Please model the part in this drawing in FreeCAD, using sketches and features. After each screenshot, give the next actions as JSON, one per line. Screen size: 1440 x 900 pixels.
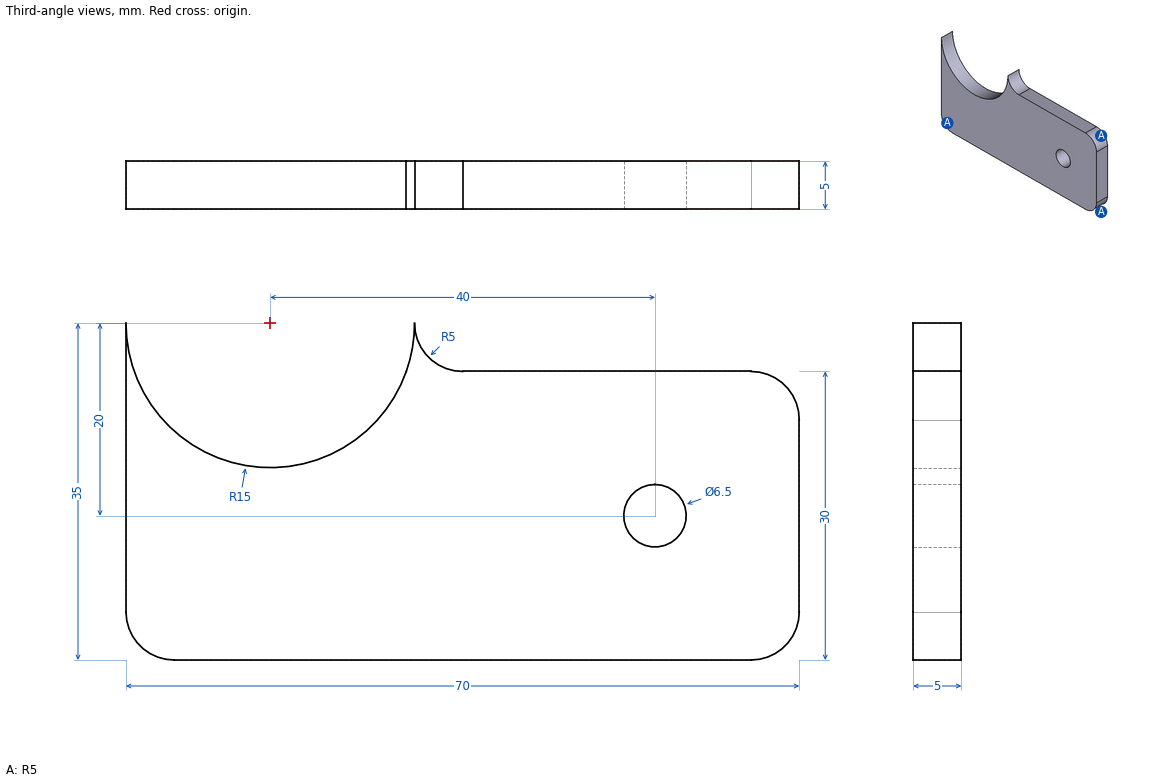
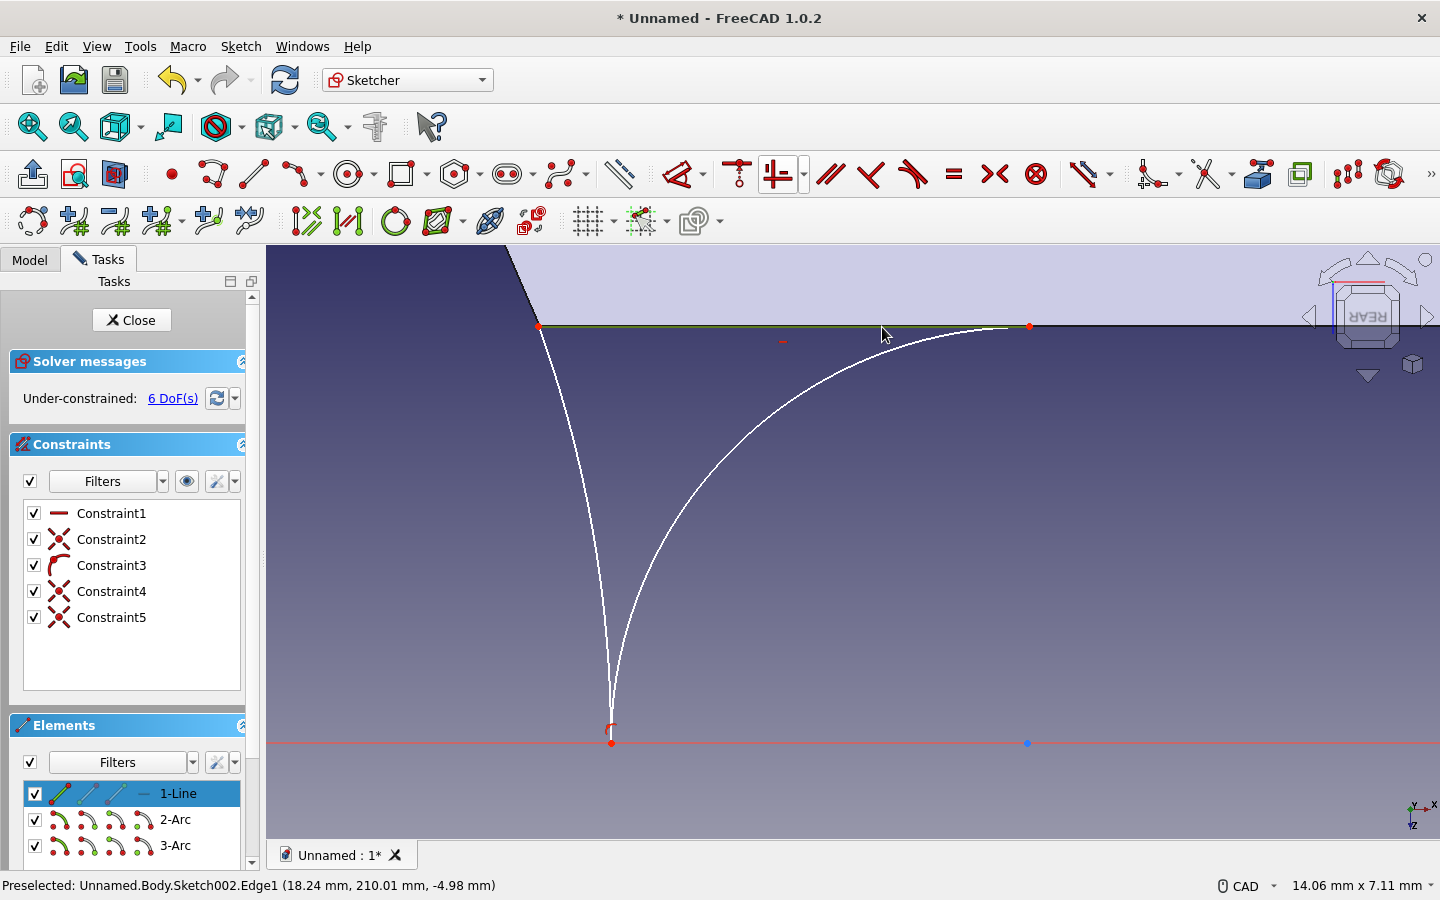
{"action": "left_click", "coordinate": [839, 372]}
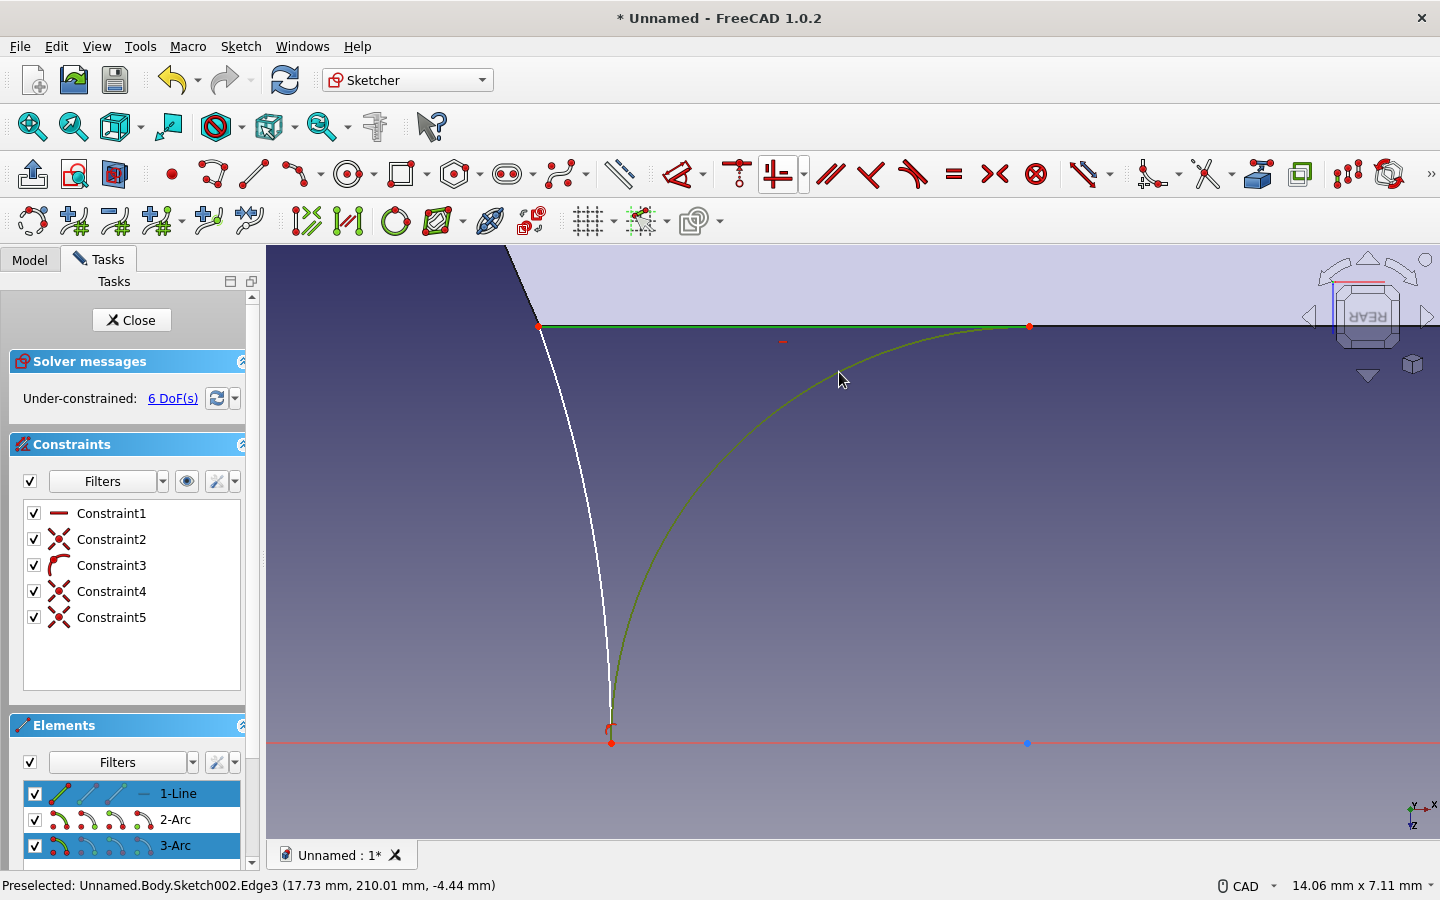
{"action": "left_click", "coordinate": [913, 174]}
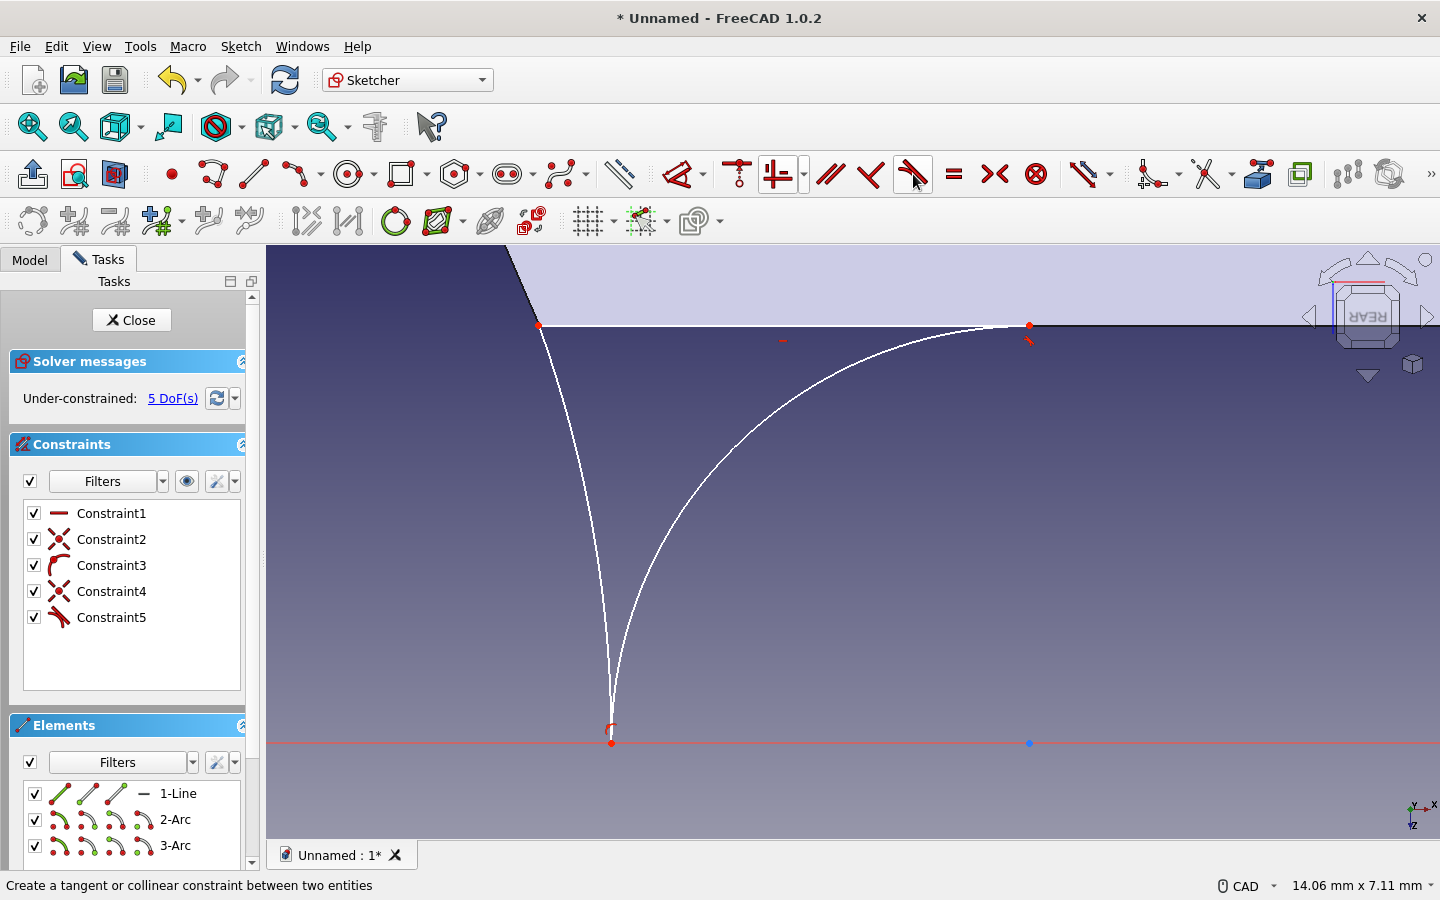
{"action": "left_click", "coordinate": [605, 616]}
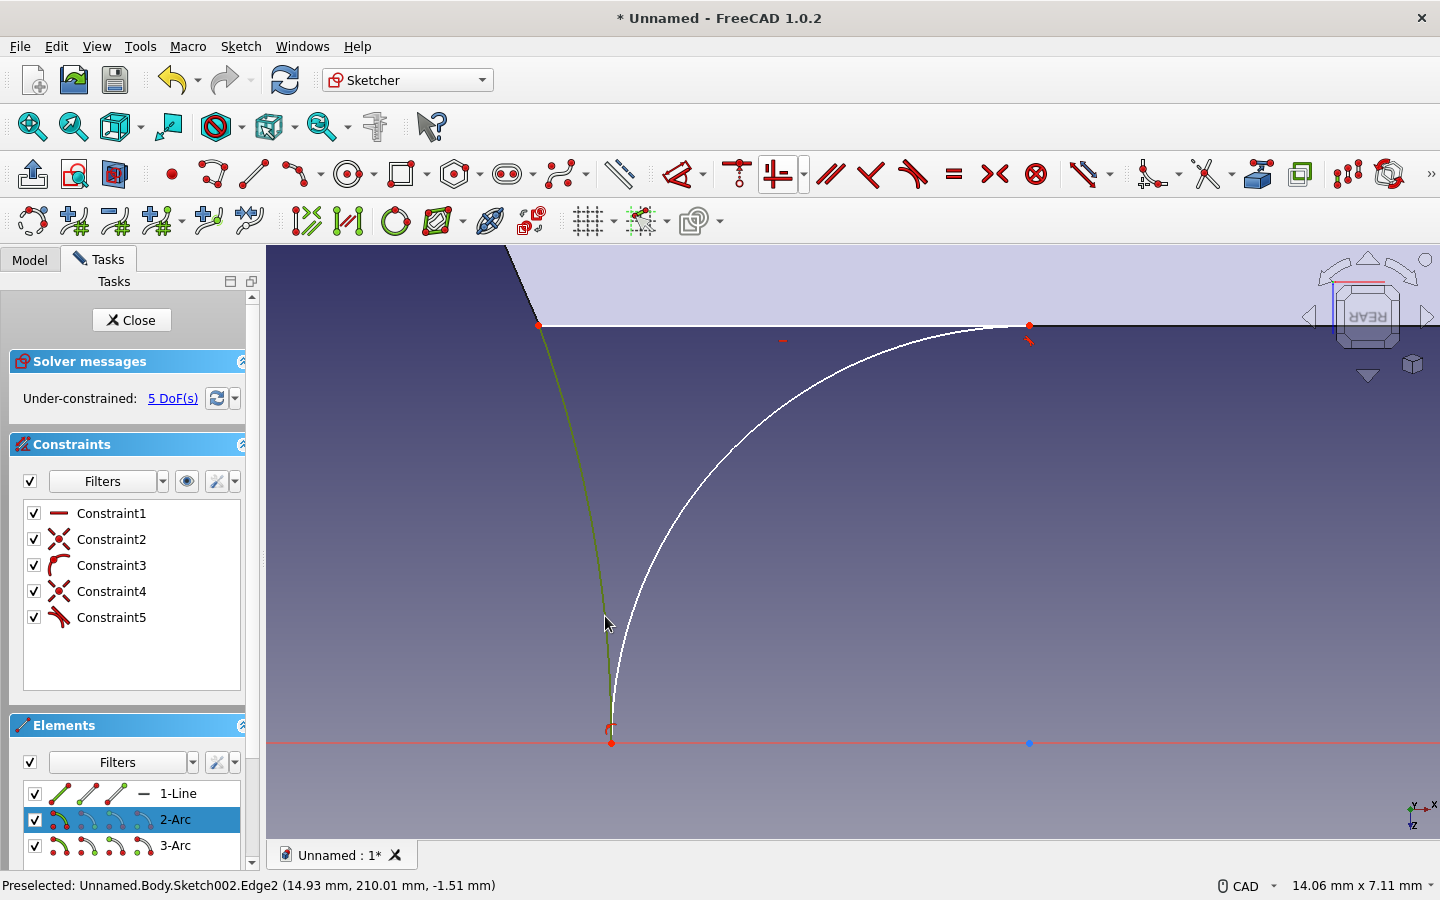
{"action": "left_click", "coordinate": [840, 371]}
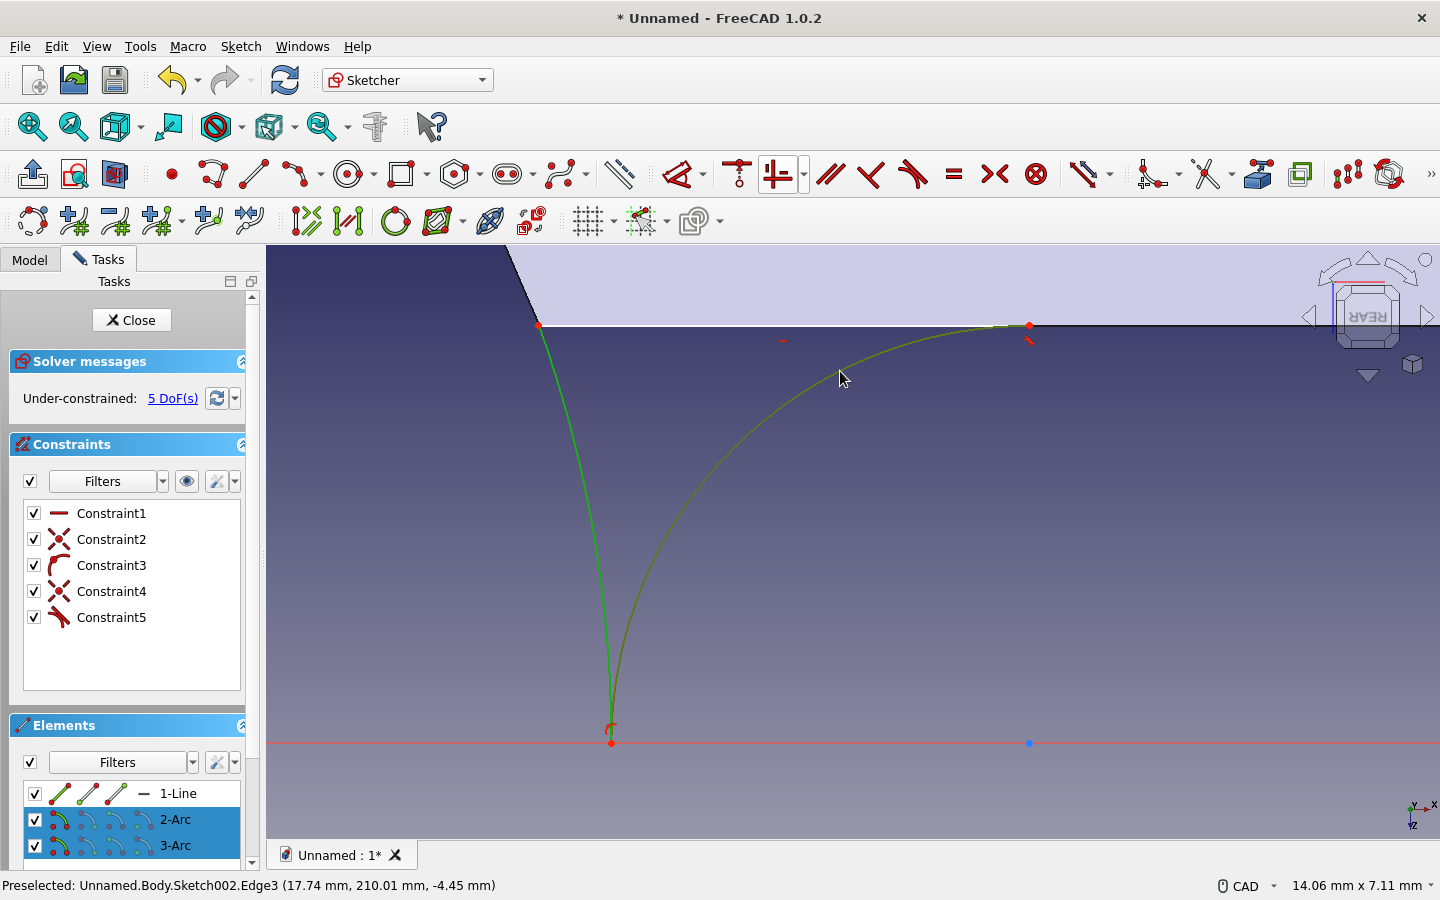
{"action": "left_click", "coordinate": [913, 174]}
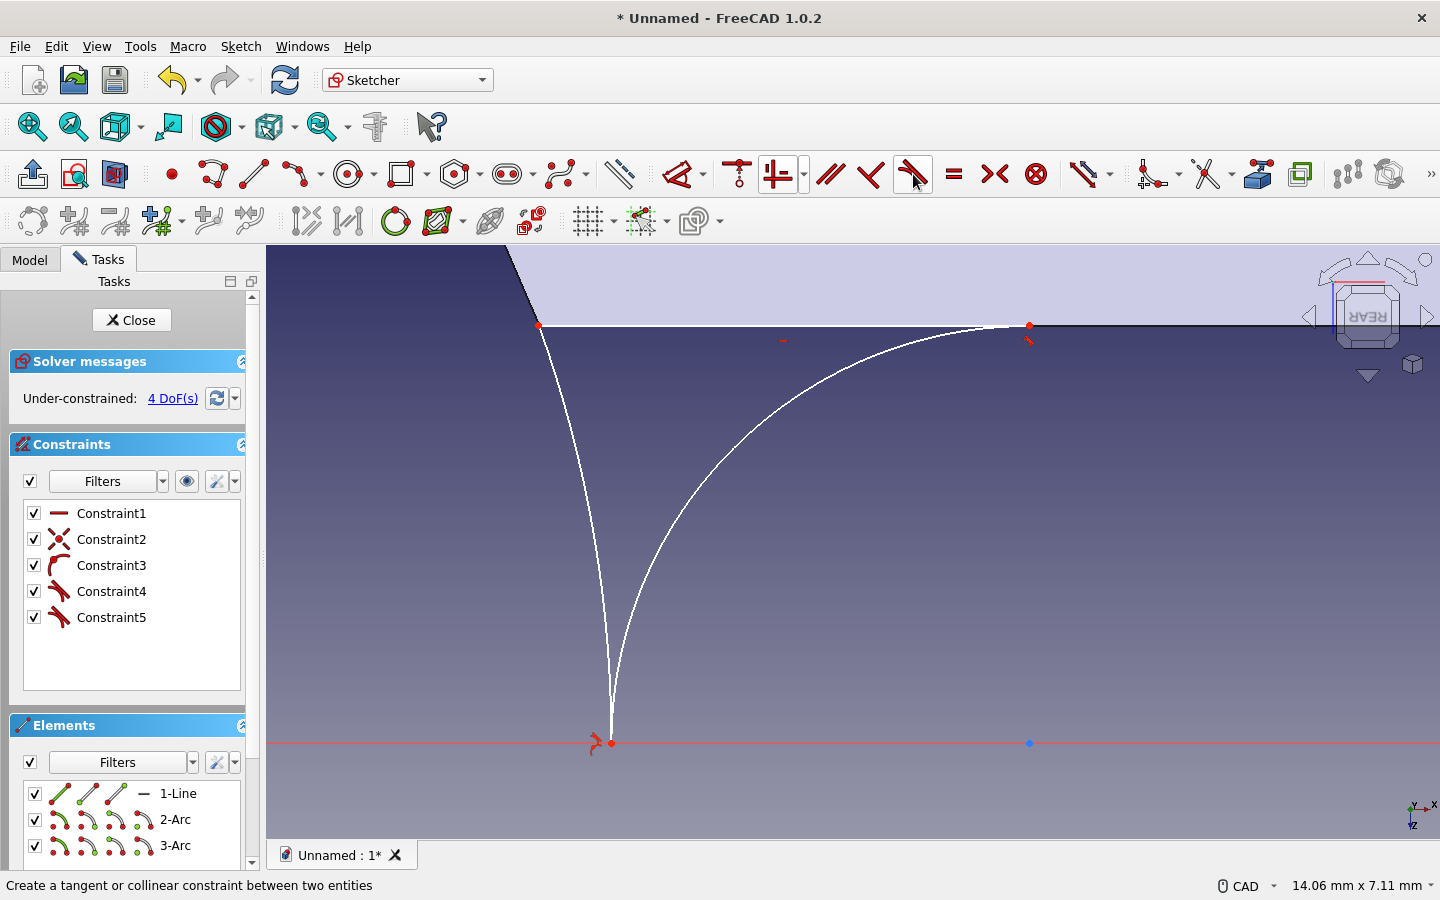
{"action": "scroll", "coordinate": [1262, 548], "scroll_direction": "down", "scroll_amount": 4}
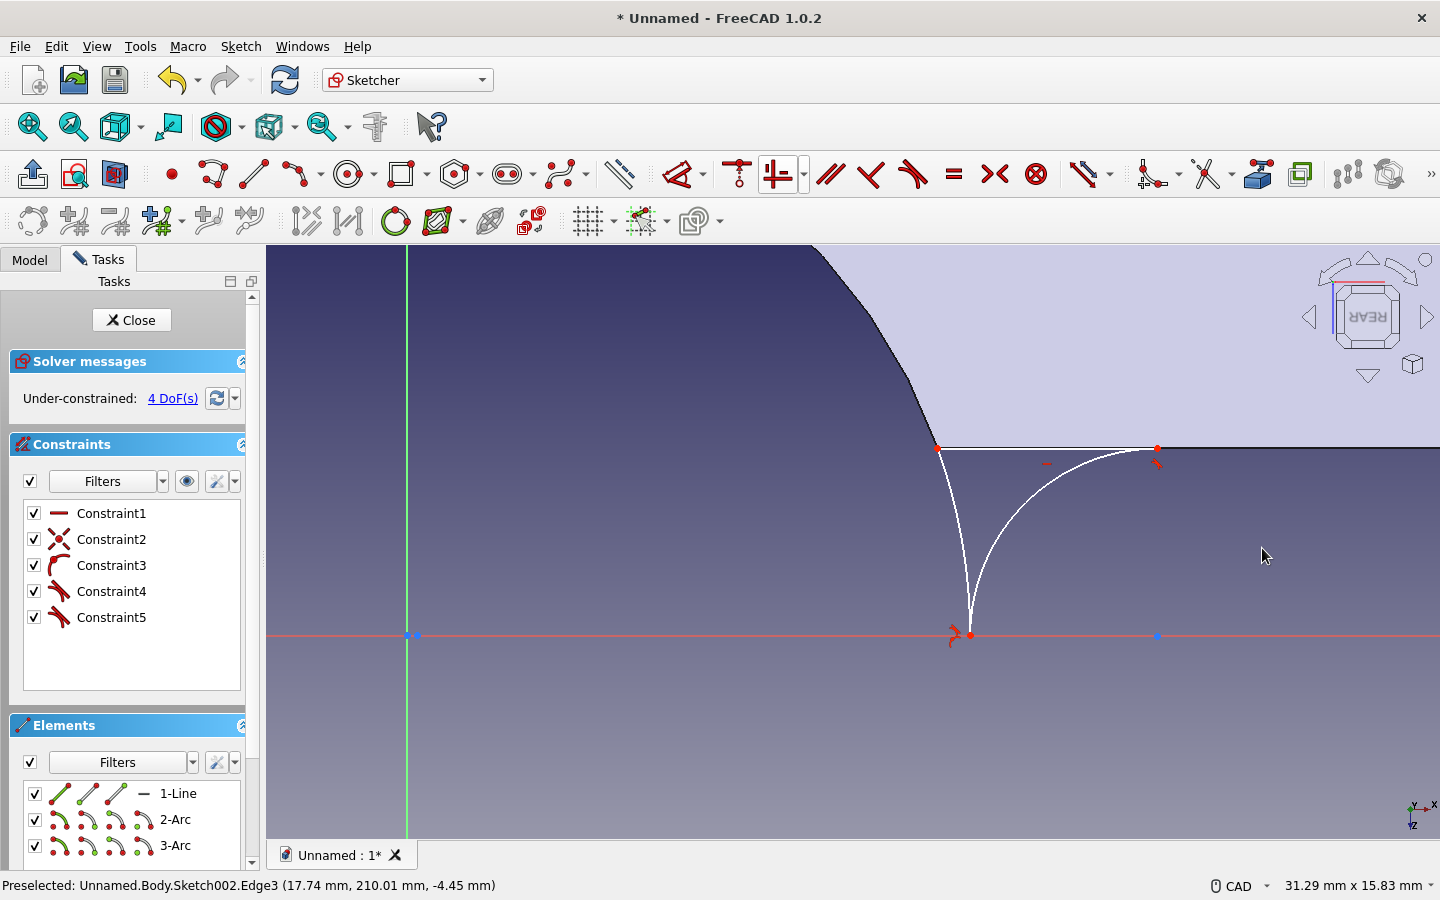
{"action": "left_click_drag", "start_coordinate": [397, 625], "coordinate": [427, 646]}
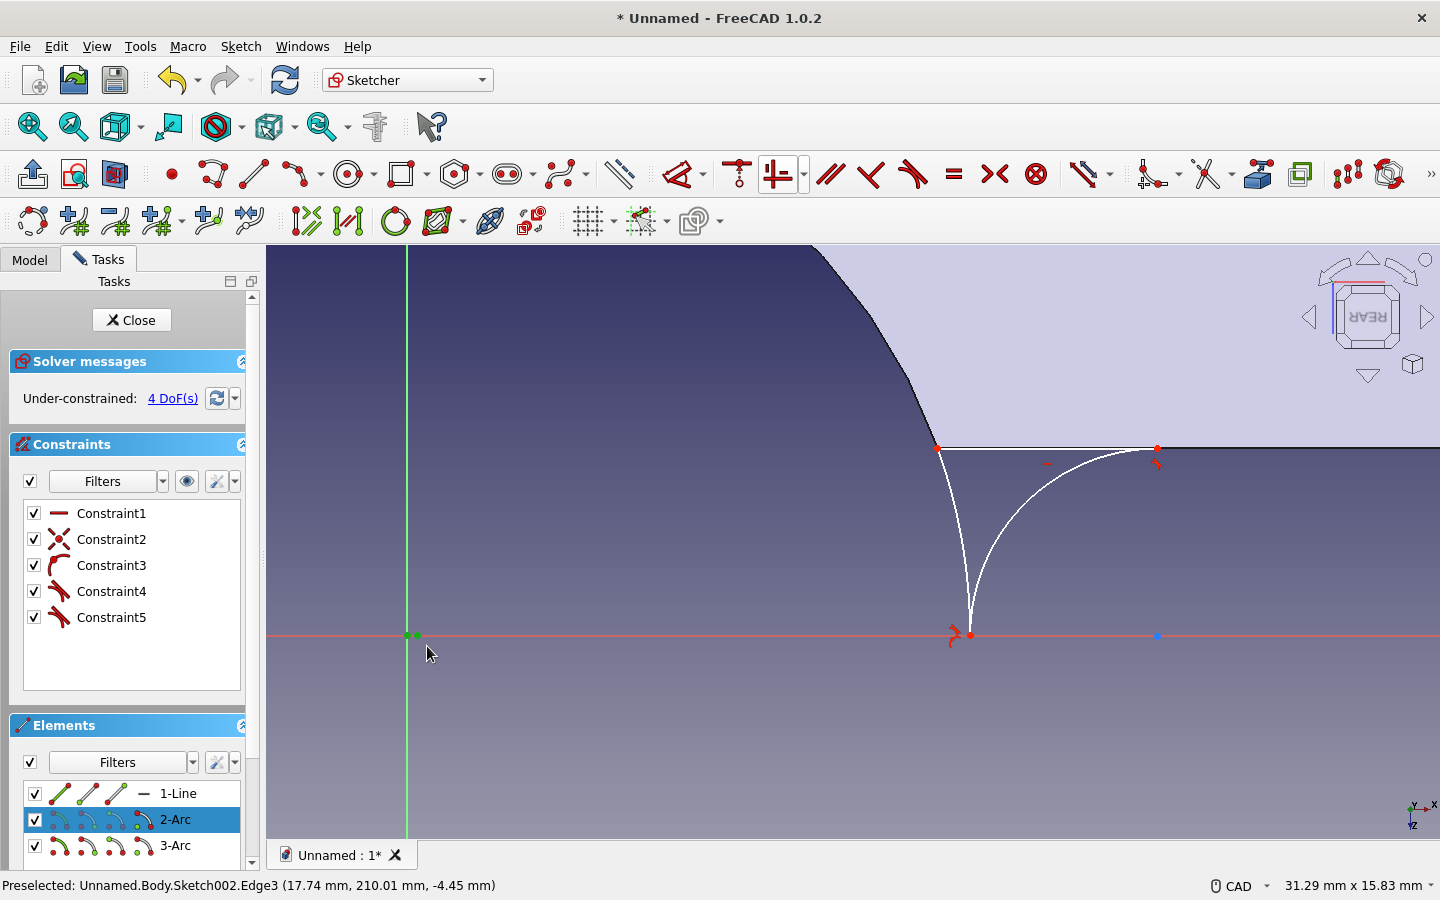
{"action": "left_click", "coordinate": [737, 174]}